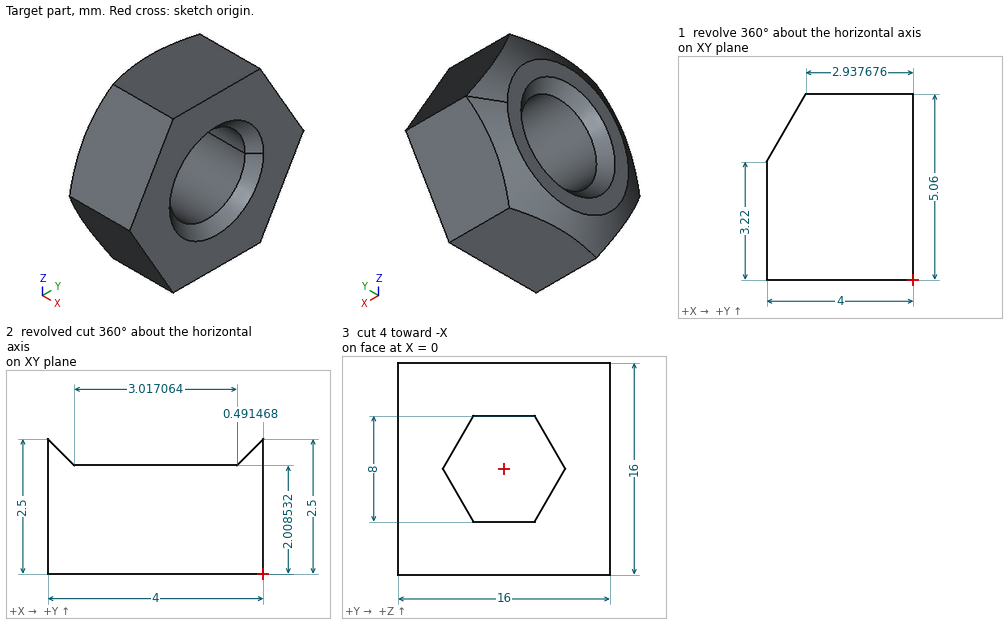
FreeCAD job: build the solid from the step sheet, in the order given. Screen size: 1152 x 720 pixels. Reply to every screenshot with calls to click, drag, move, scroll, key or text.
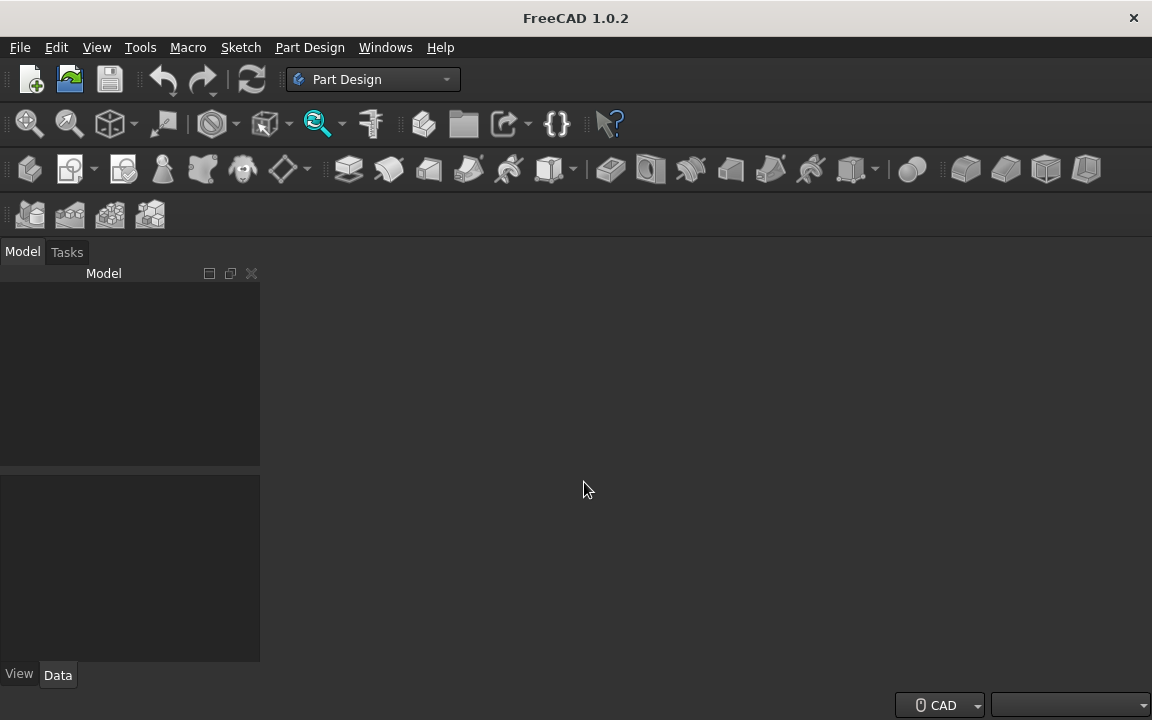
key(ctrl+n)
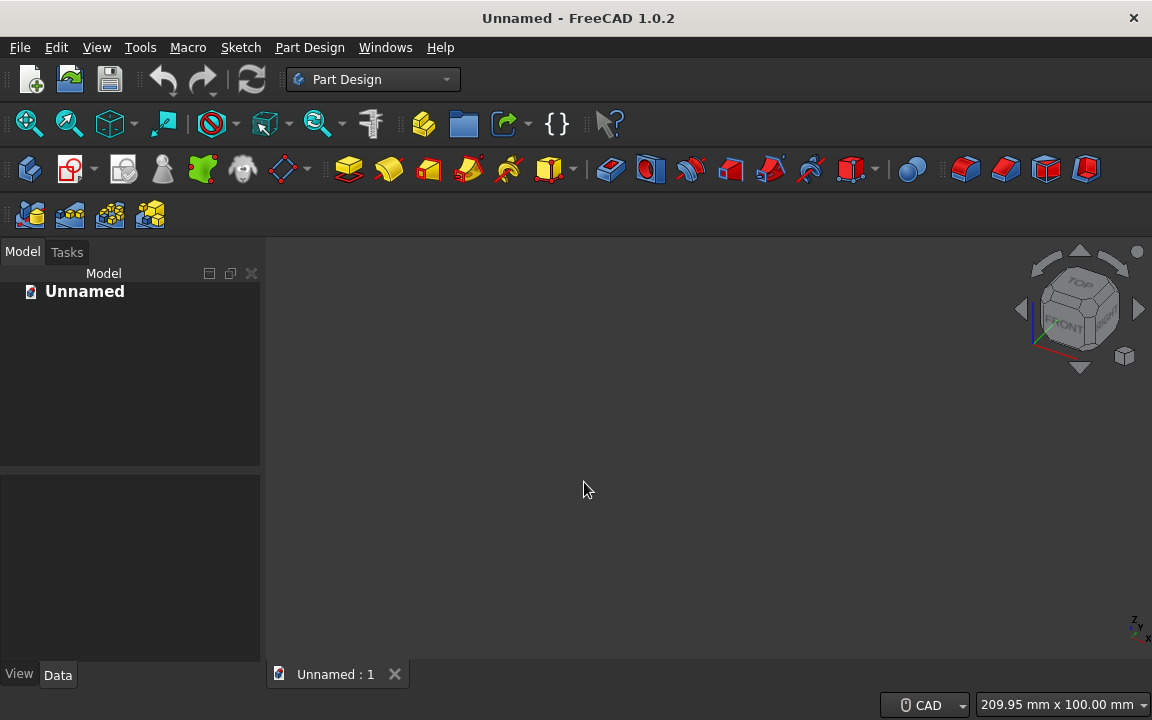
click(70, 170)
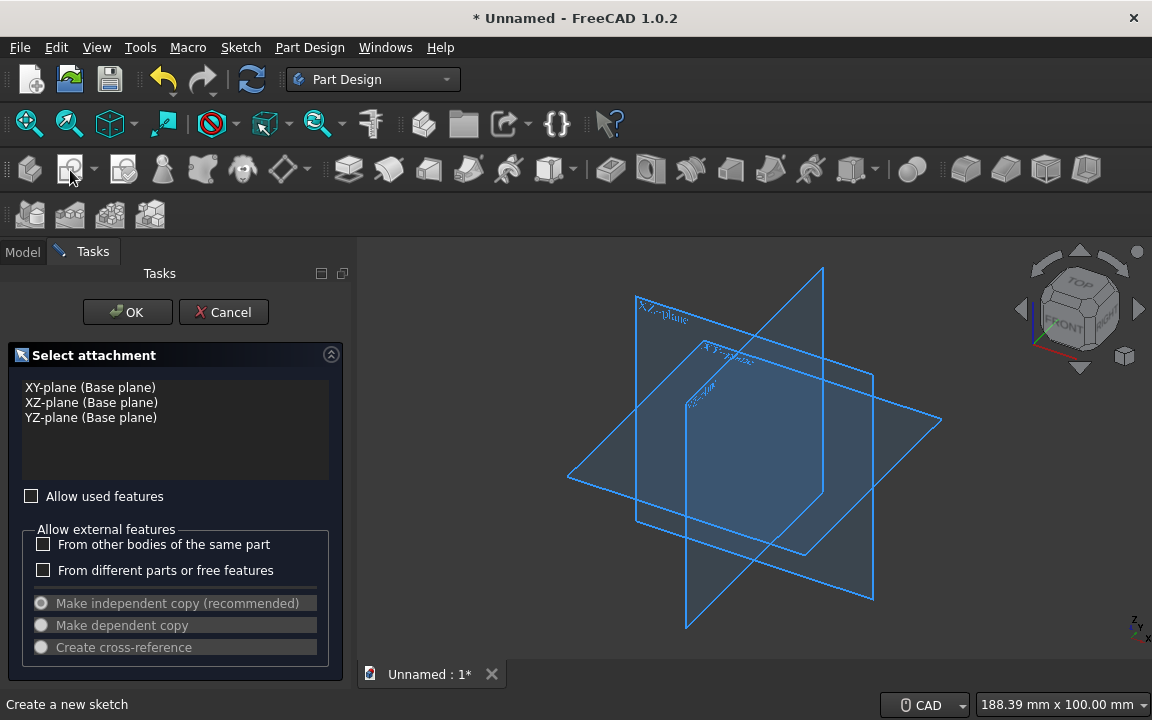
click(82, 388)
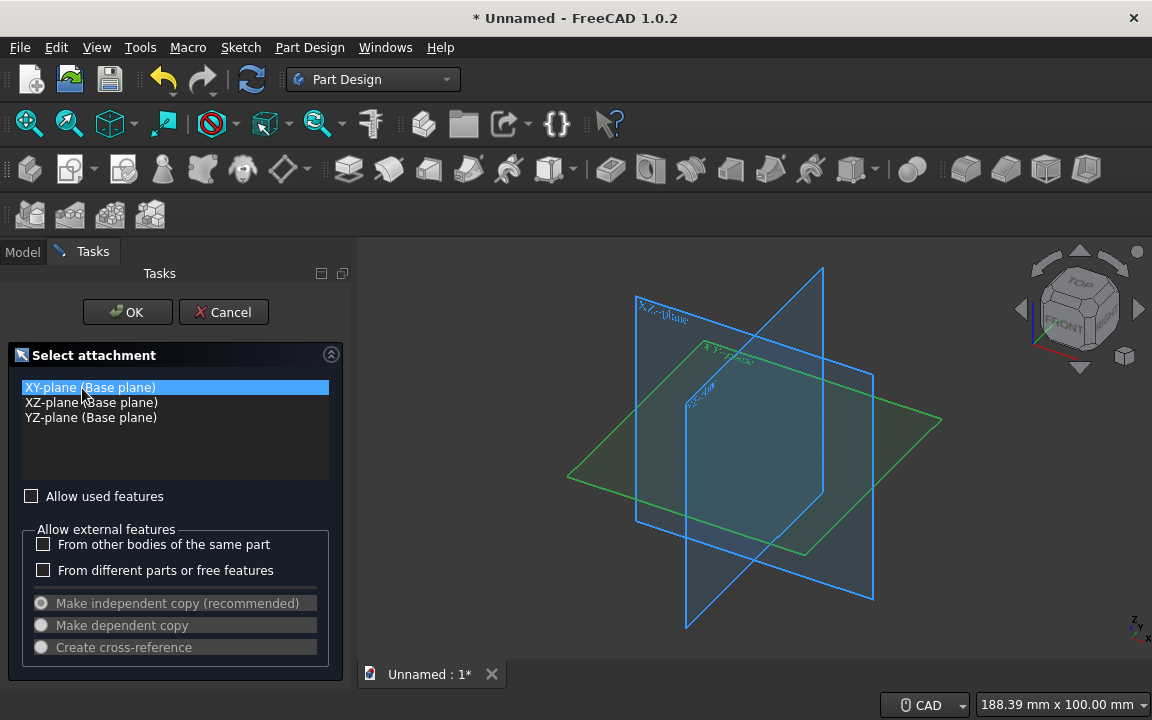
click(128, 312)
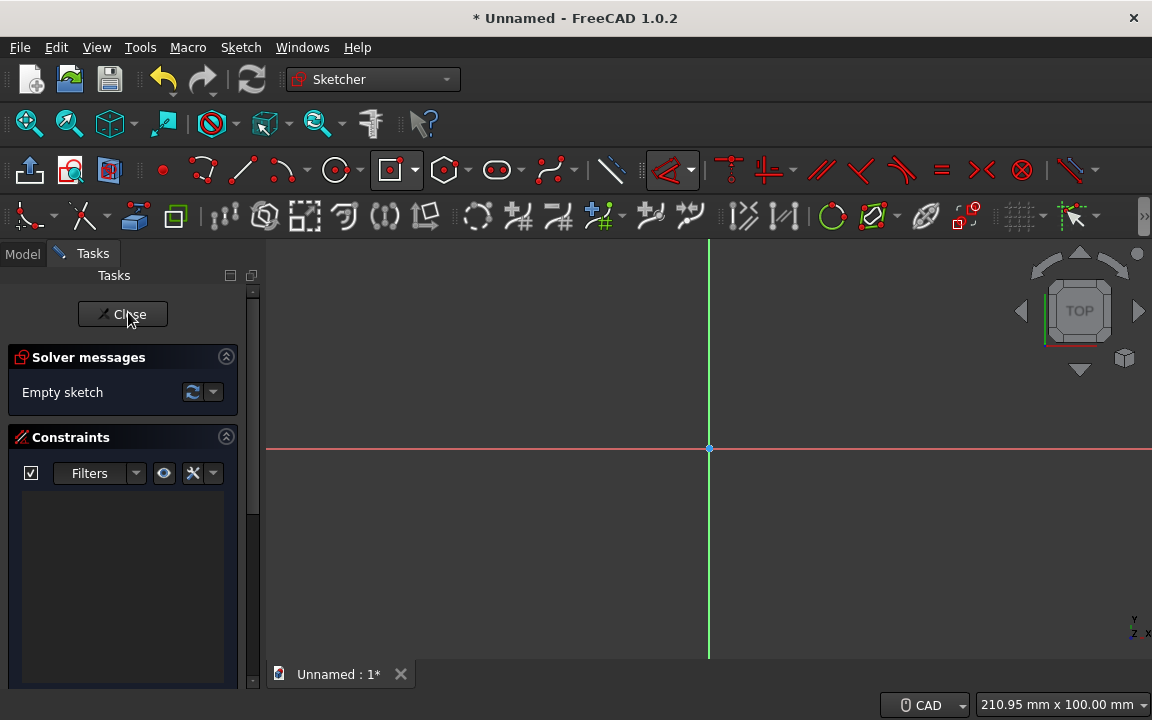
scroll(707, 437, up, 12)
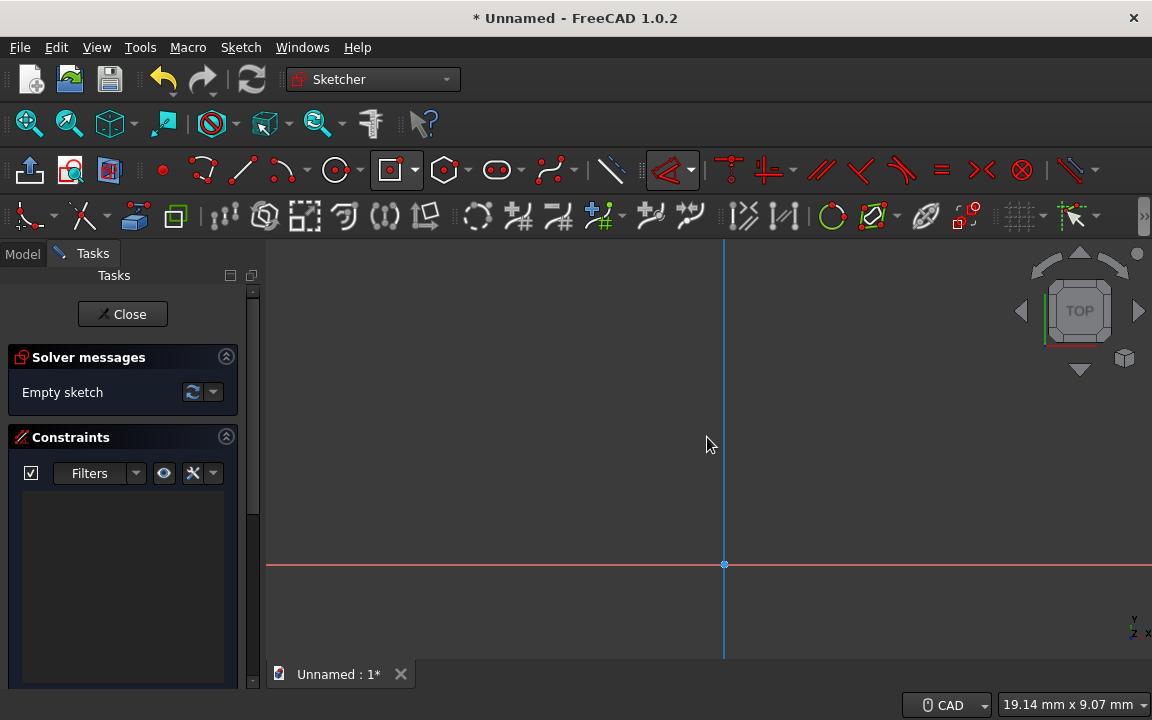
key(g)
key(m)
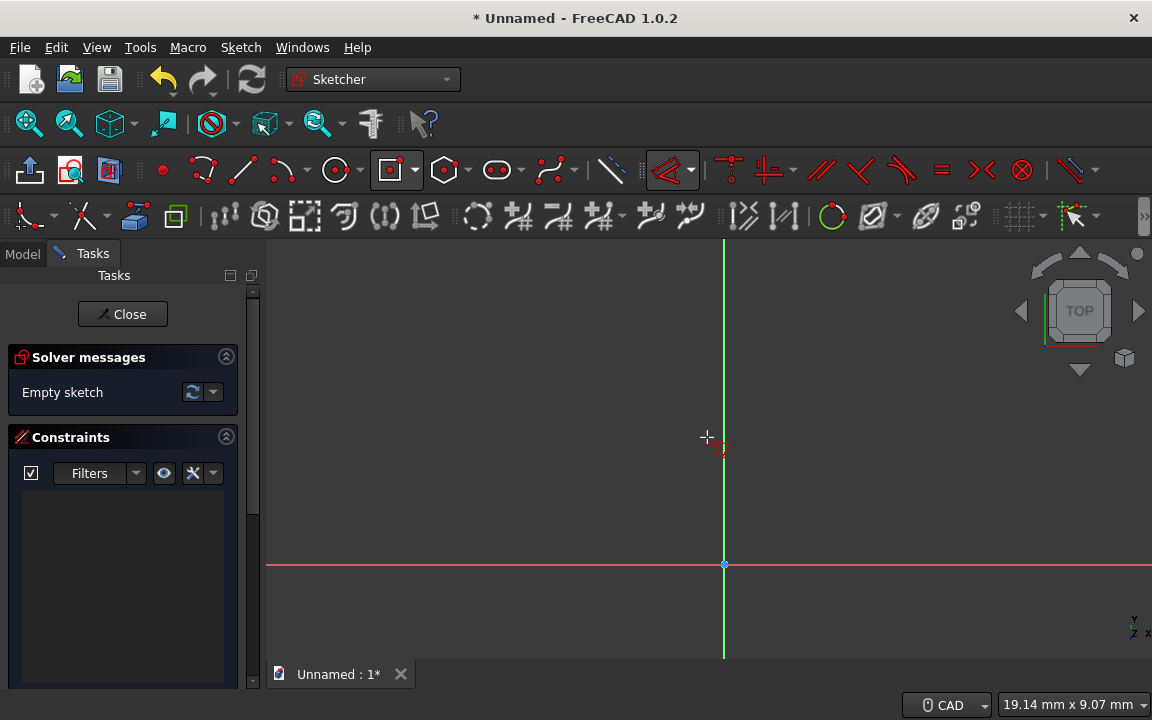
click(724, 565)
click(715, 330)
click(588, 330)
click(539, 415)
click(539, 556)
click(724, 565)
key(Escape)
key(Escape)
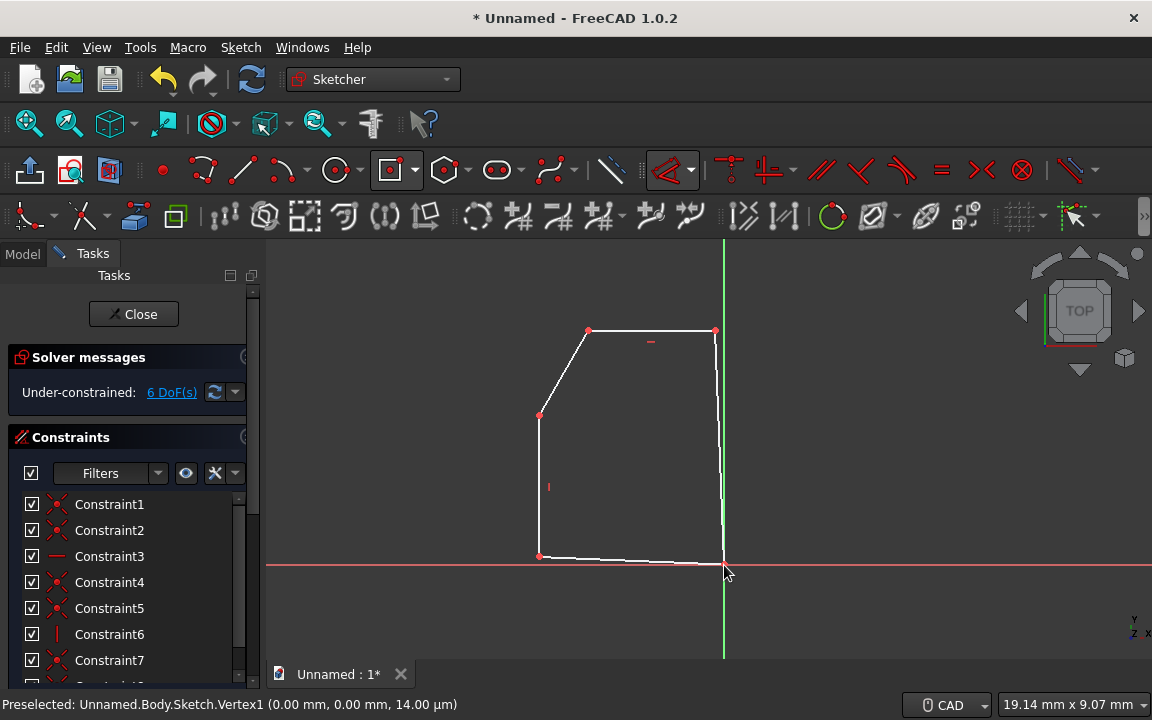
click(721, 494)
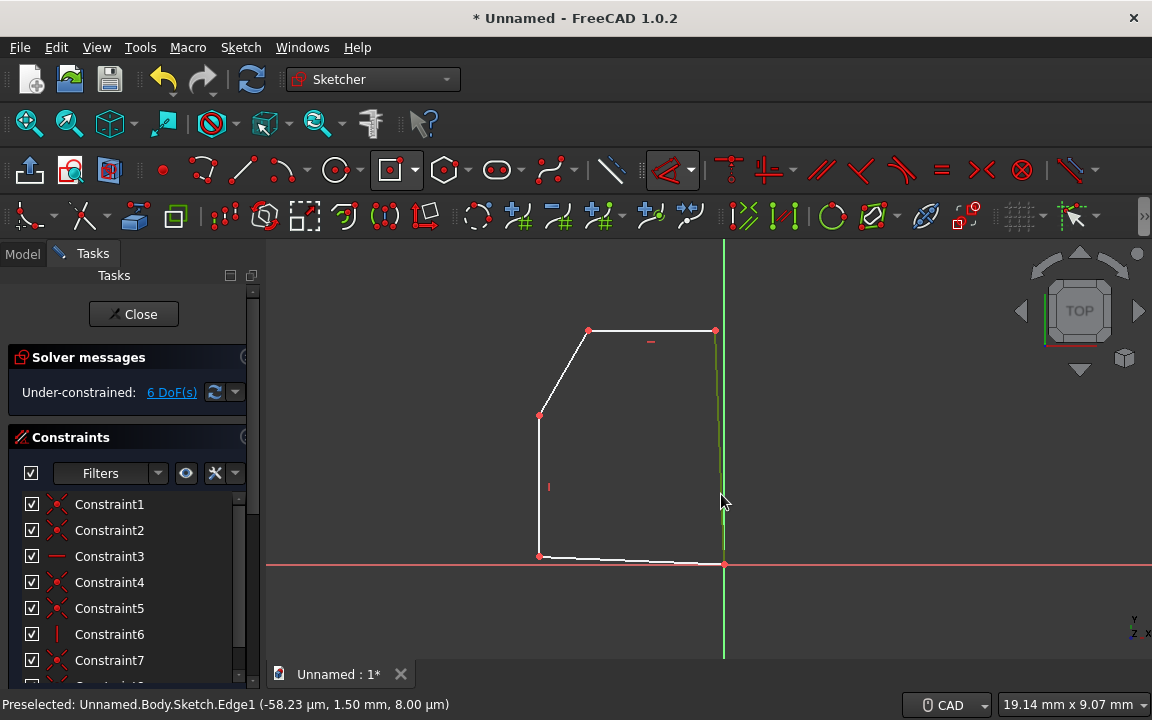
key(v)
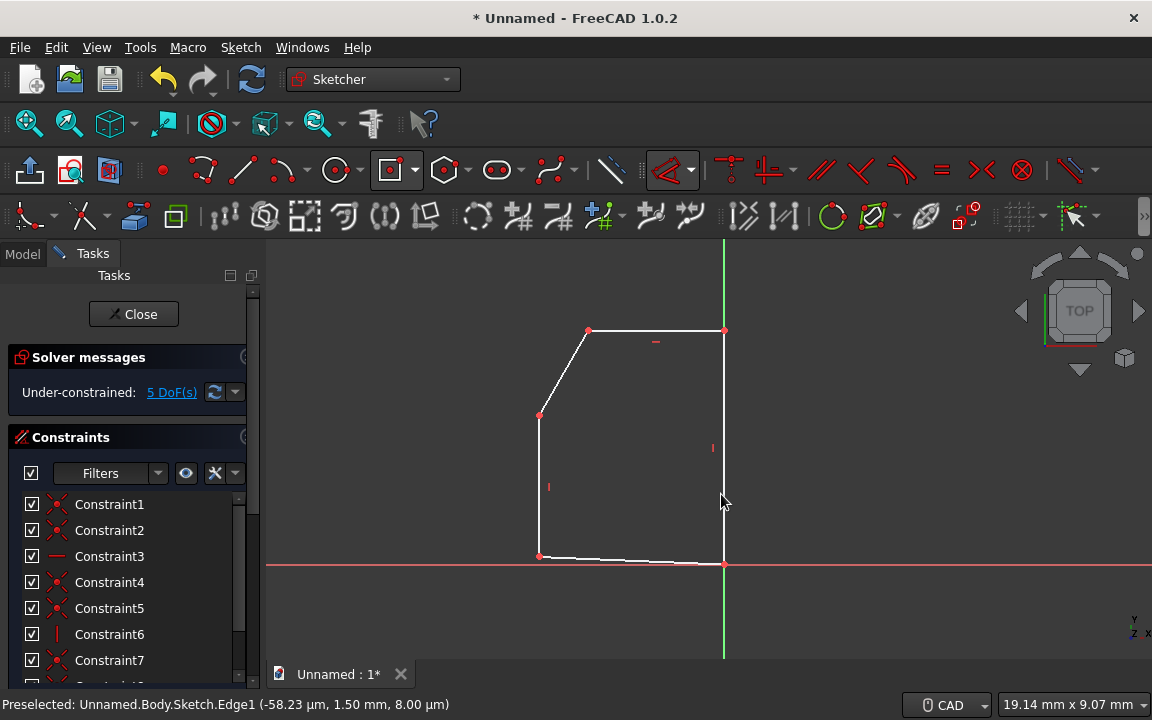
click(669, 562)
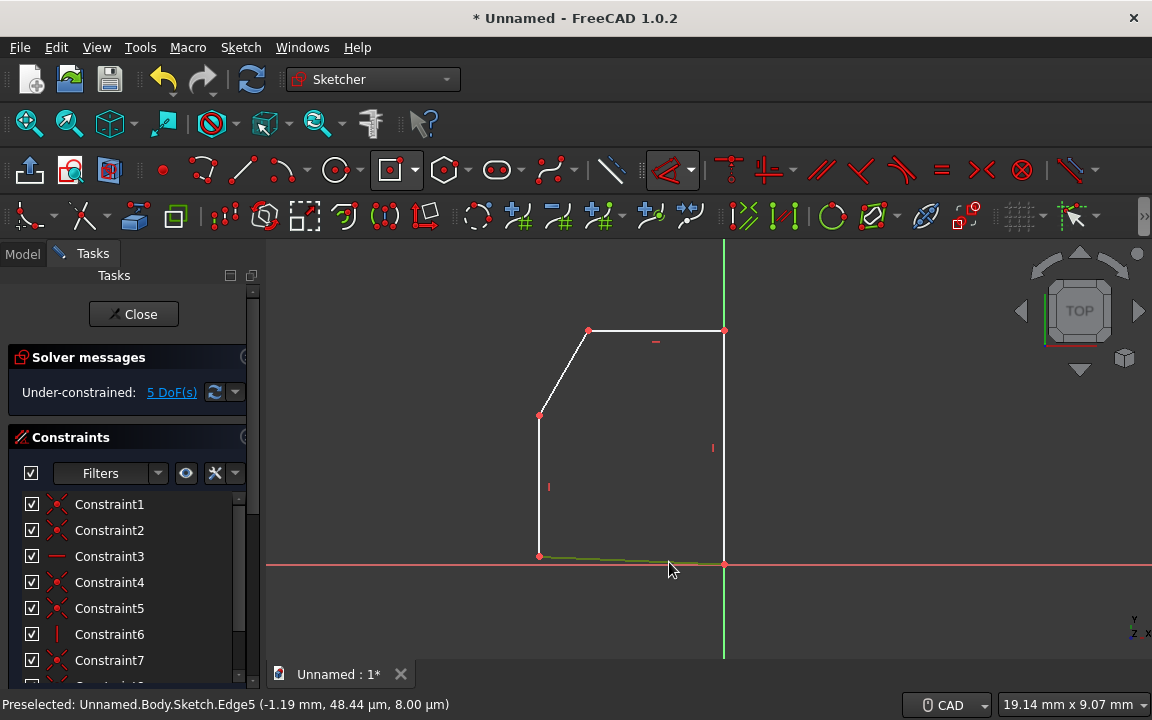
key(h)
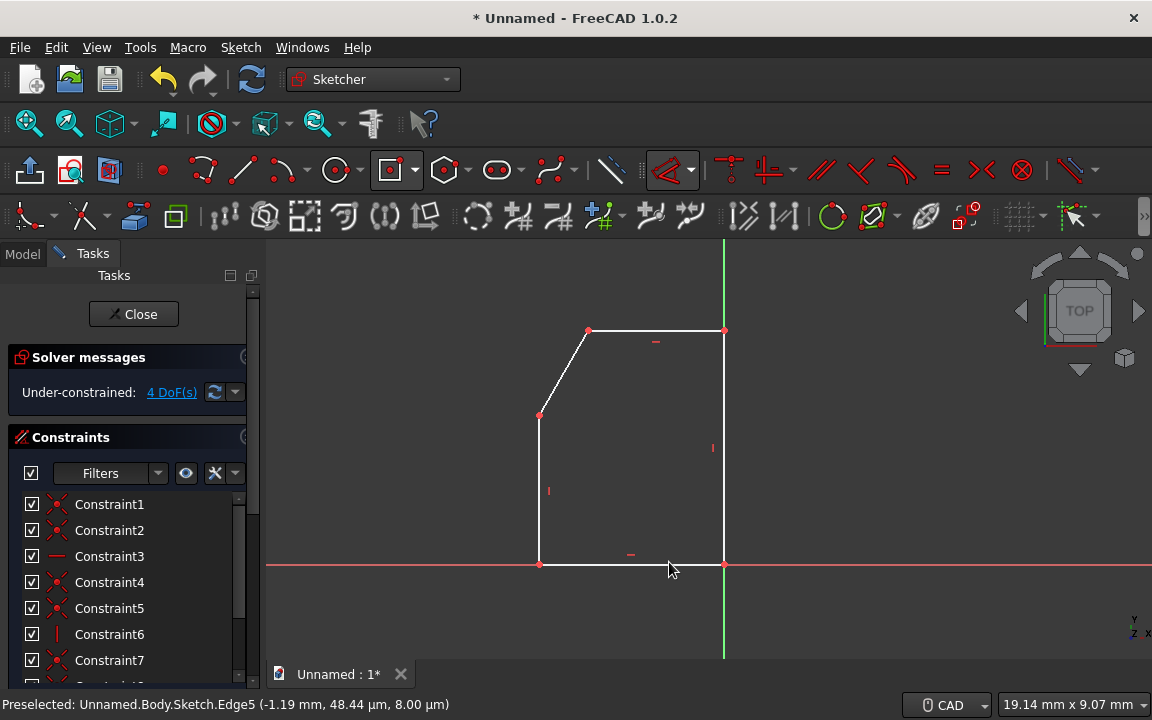
click(595, 565)